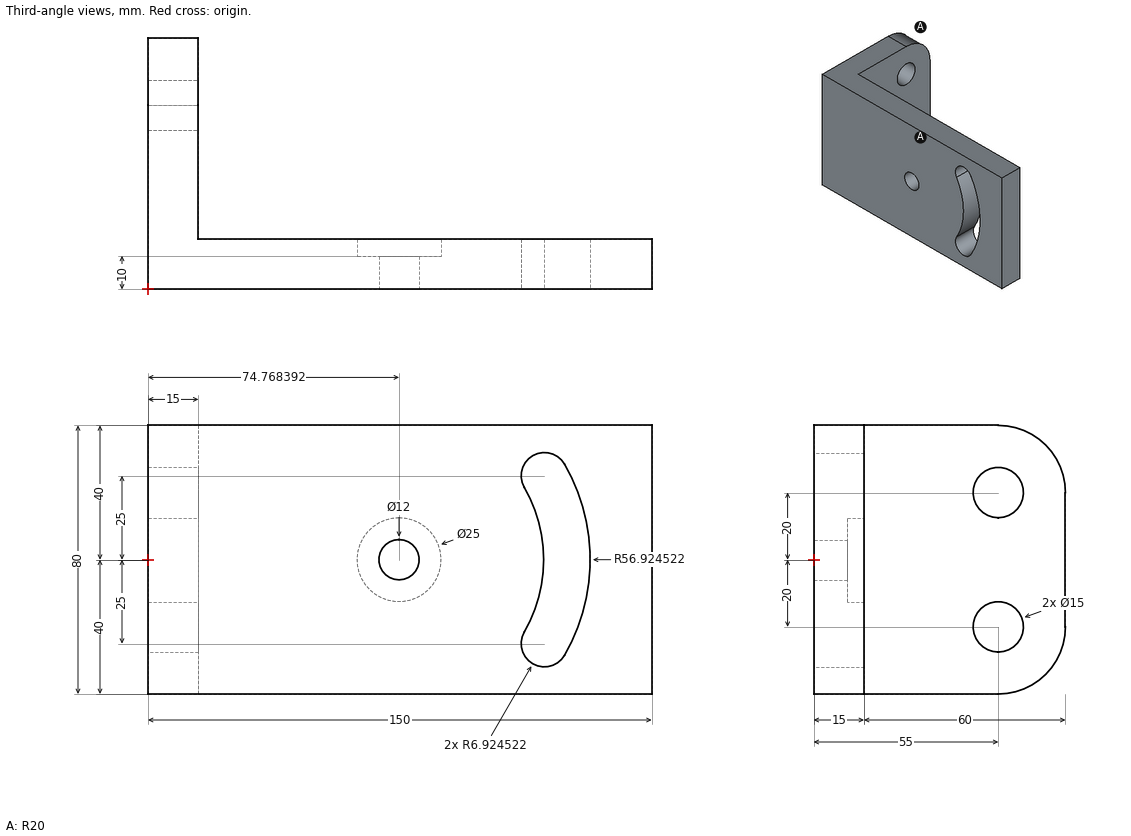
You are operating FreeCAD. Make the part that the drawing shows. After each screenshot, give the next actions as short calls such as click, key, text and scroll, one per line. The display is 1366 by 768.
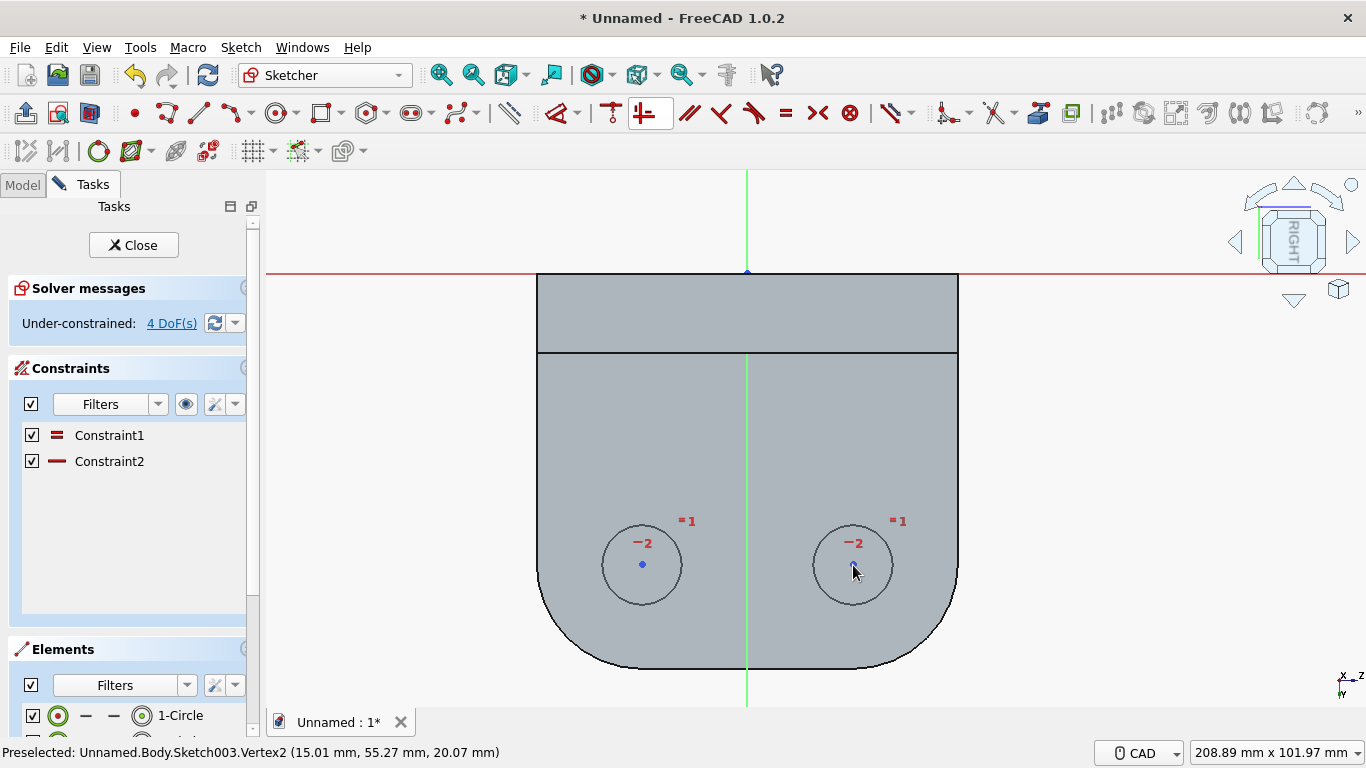
click(556, 114)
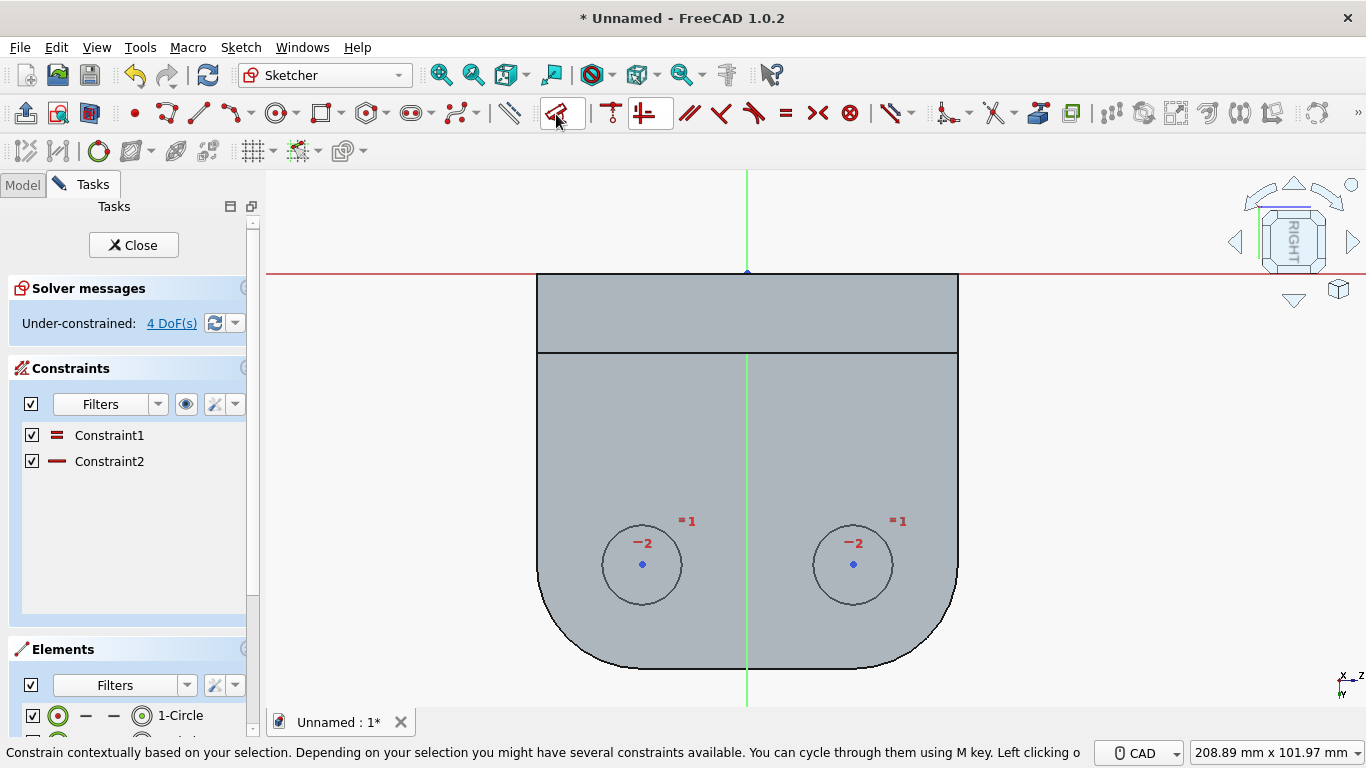
click(670, 537)
click(693, 514)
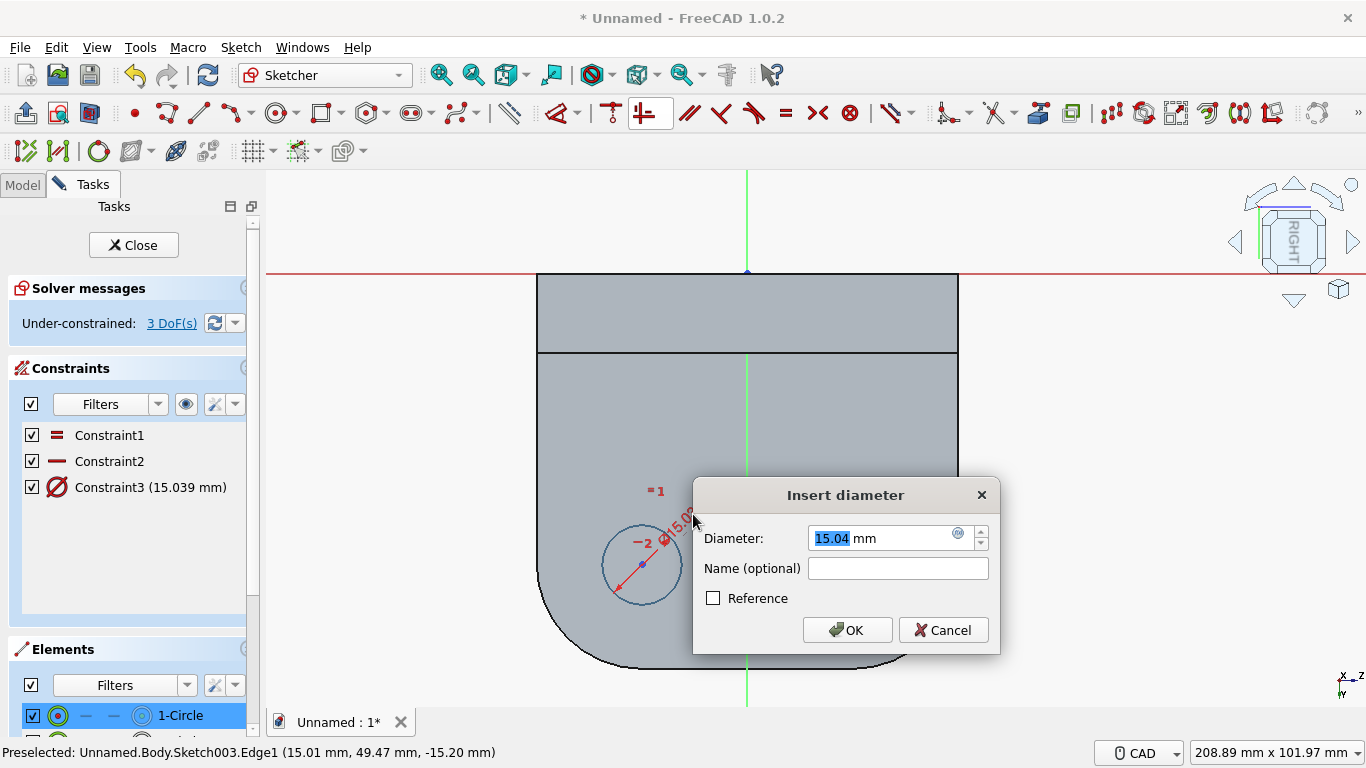
text(15)
key(Return)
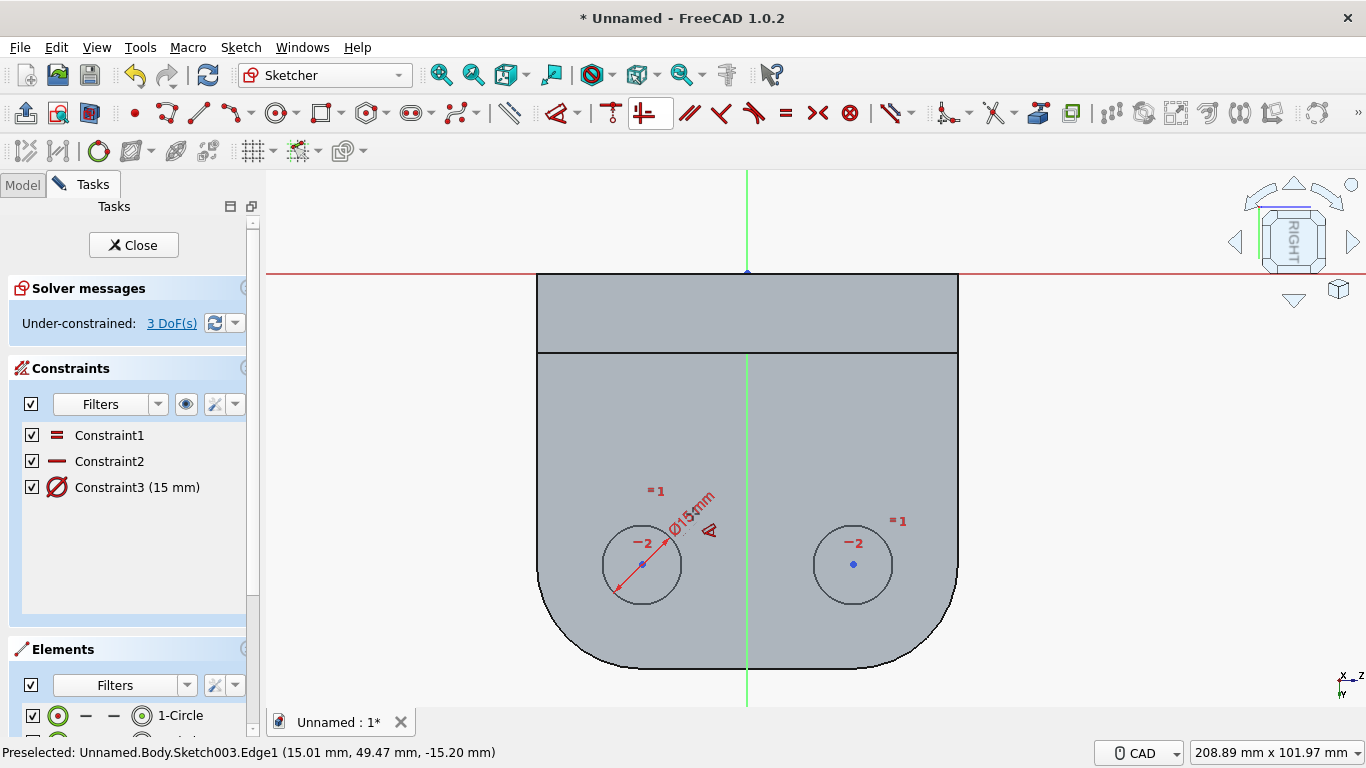
click(642, 565)
click(695, 240)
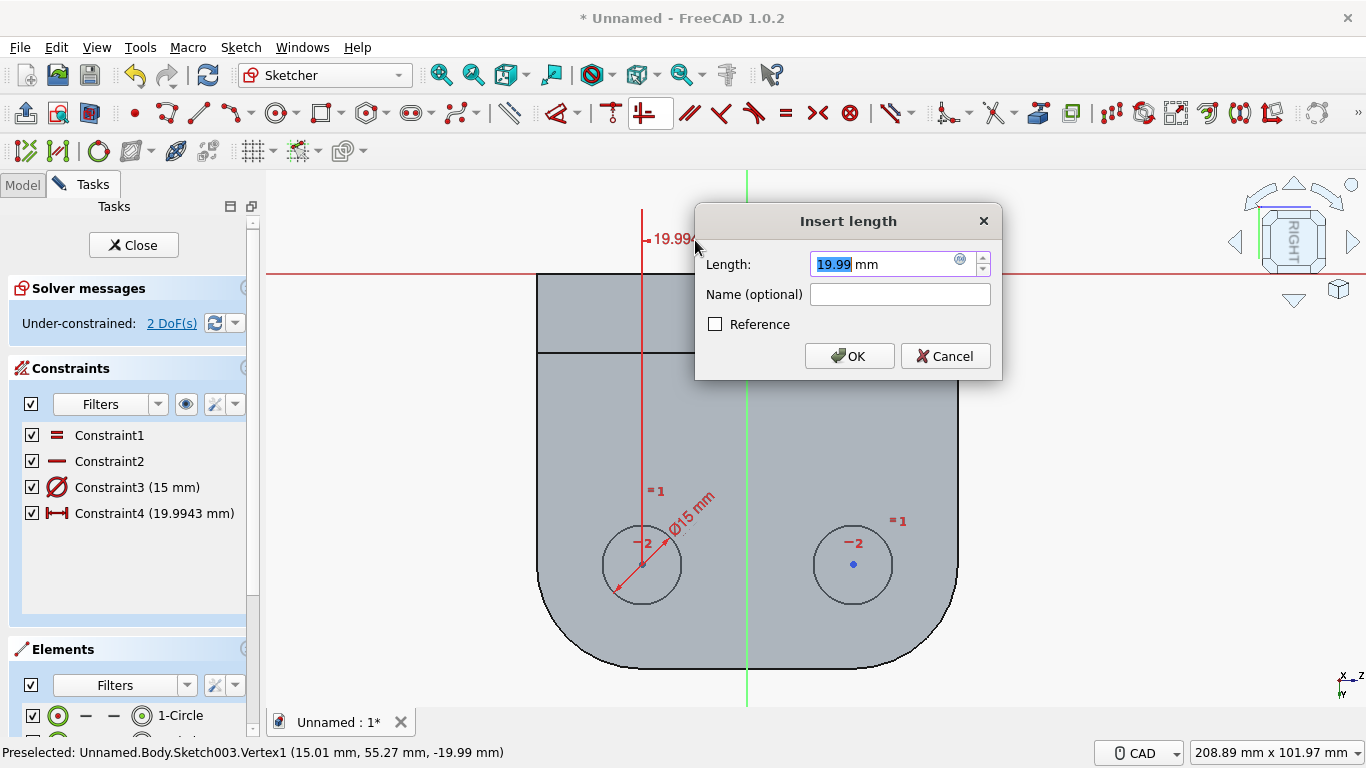
text(20)
key(Return)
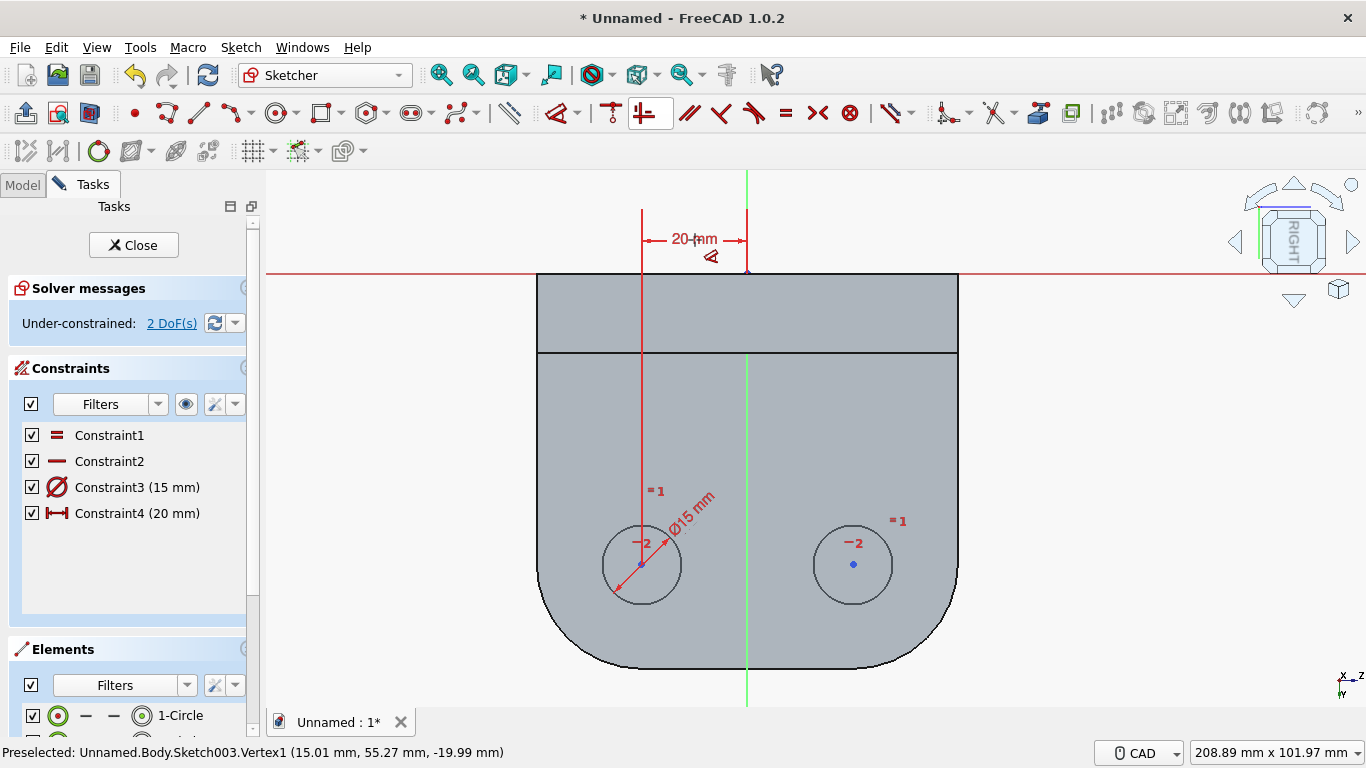
click(642, 565)
click(608, 419)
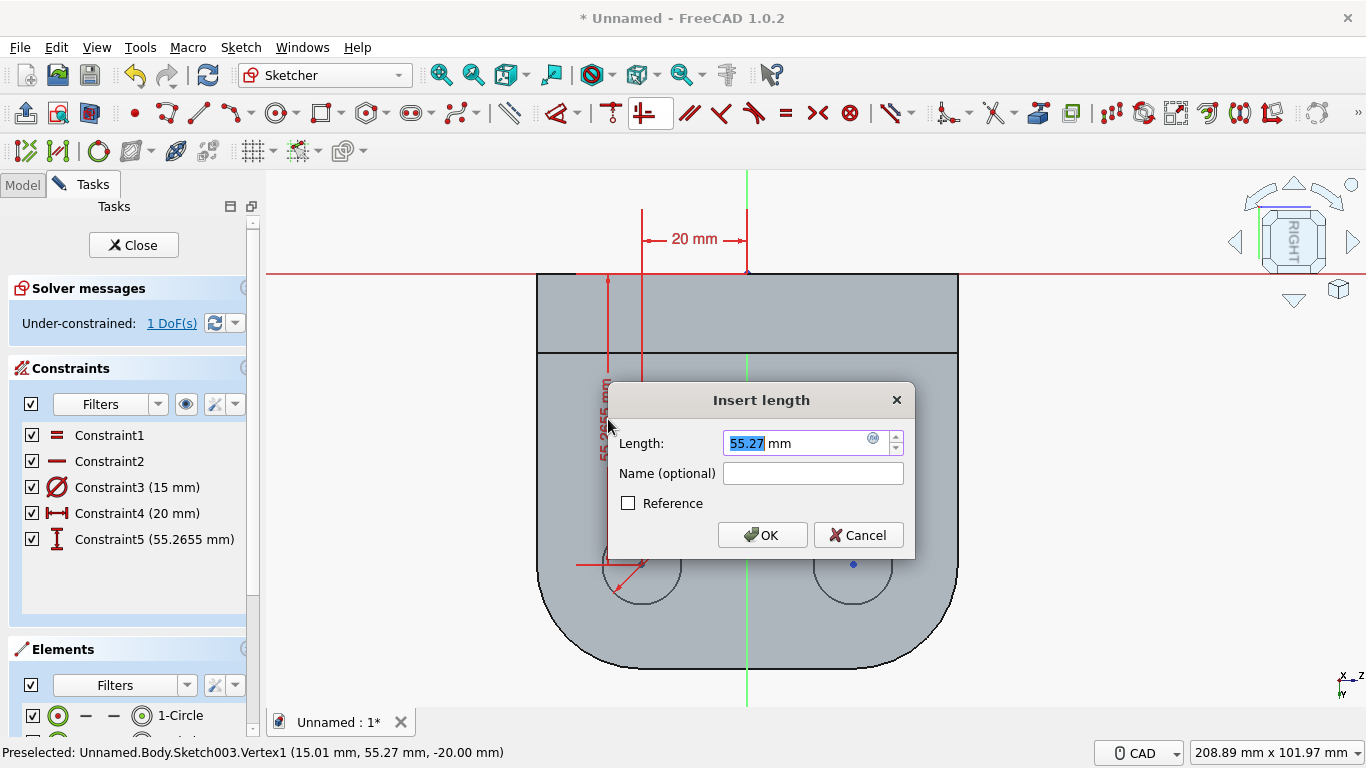
text(55)
key(Return)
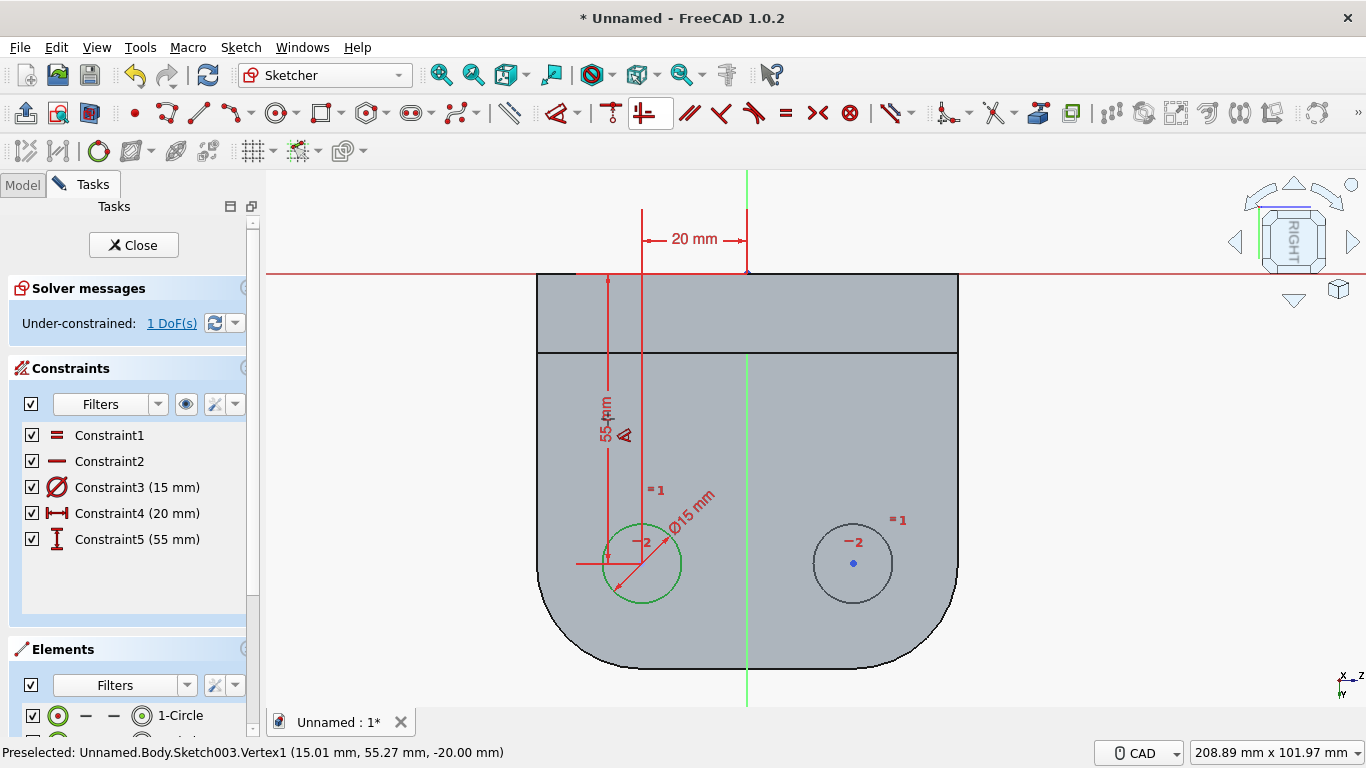
click(853, 564)
click(800, 240)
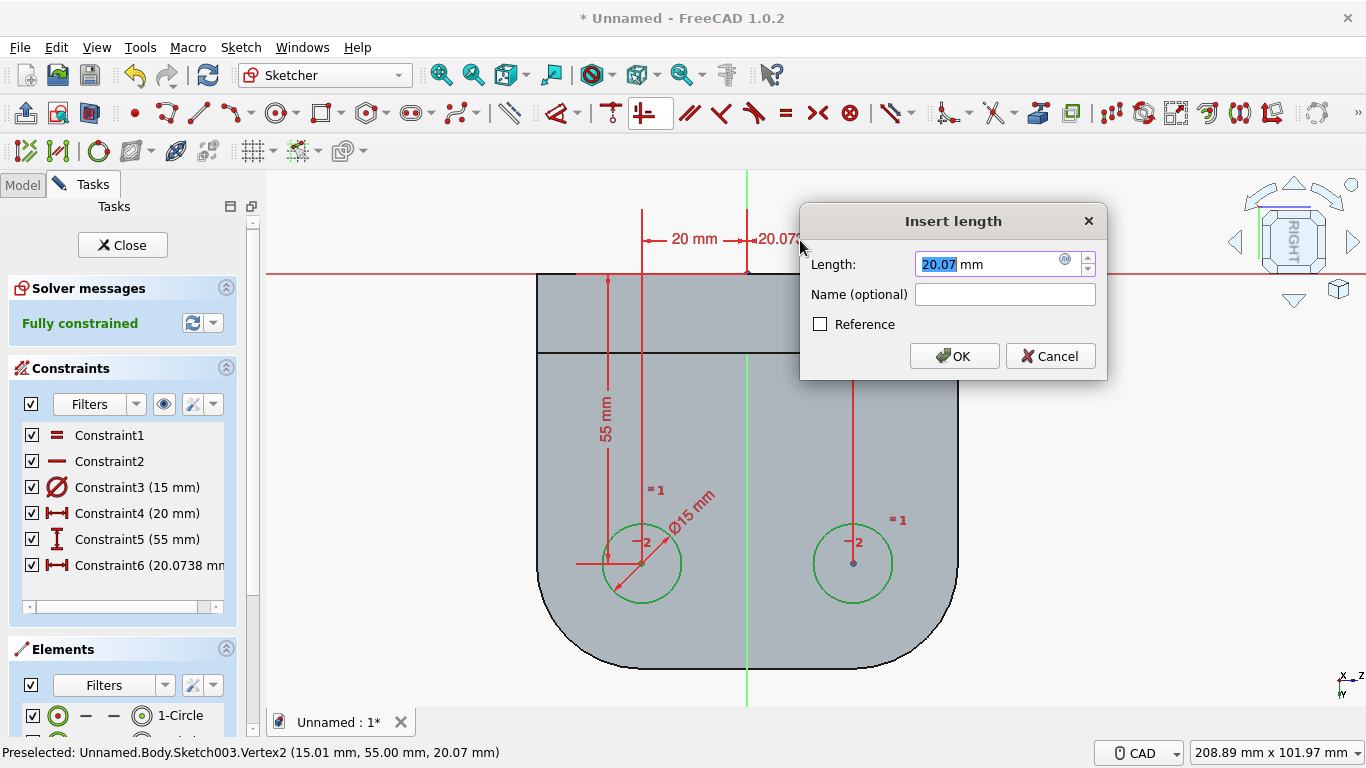
text(20)
key(Return)
key(Escape)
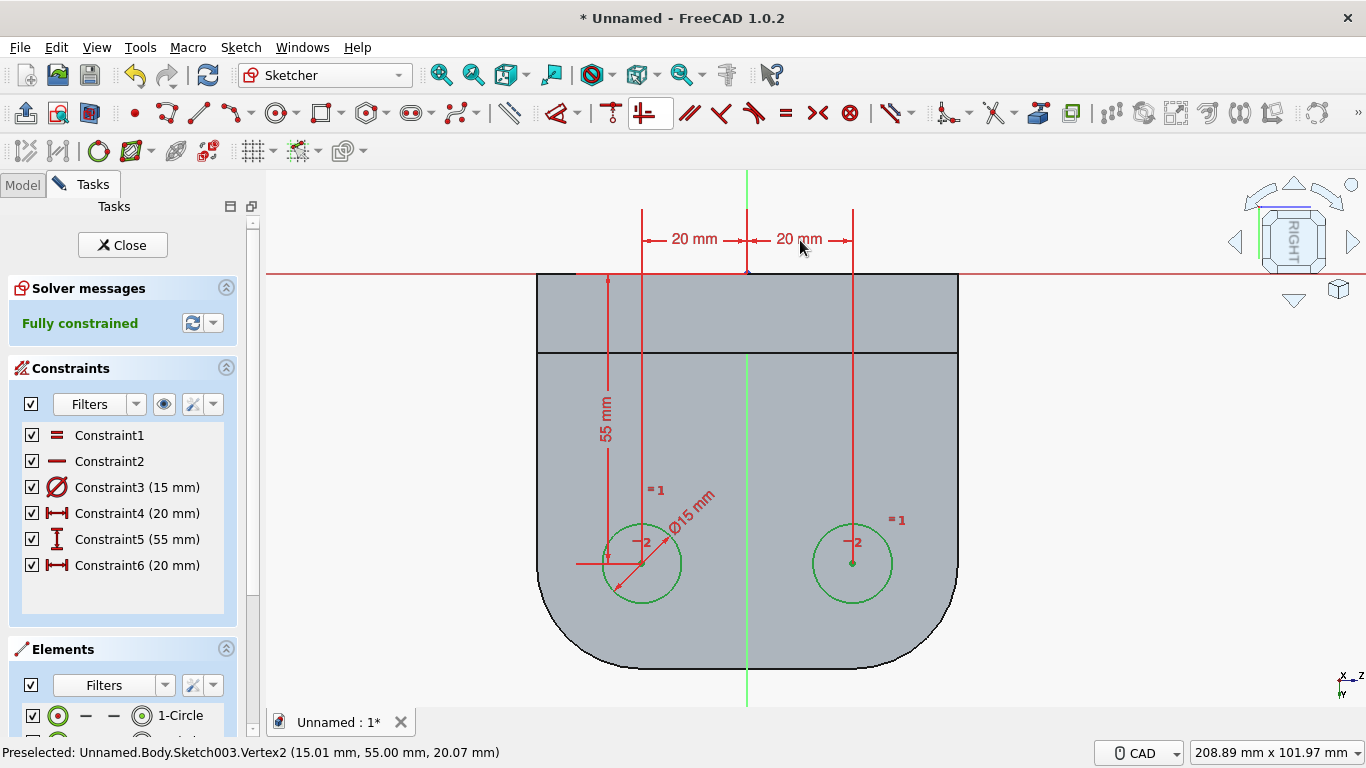
click(123, 245)